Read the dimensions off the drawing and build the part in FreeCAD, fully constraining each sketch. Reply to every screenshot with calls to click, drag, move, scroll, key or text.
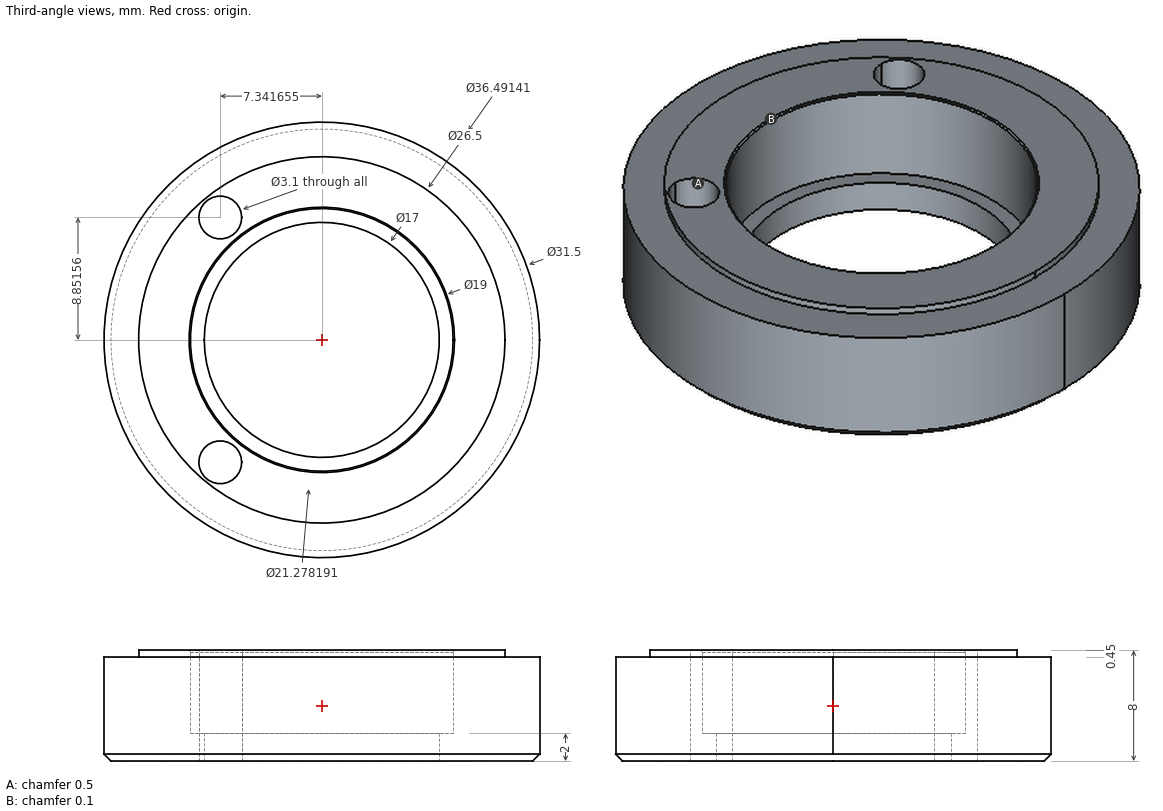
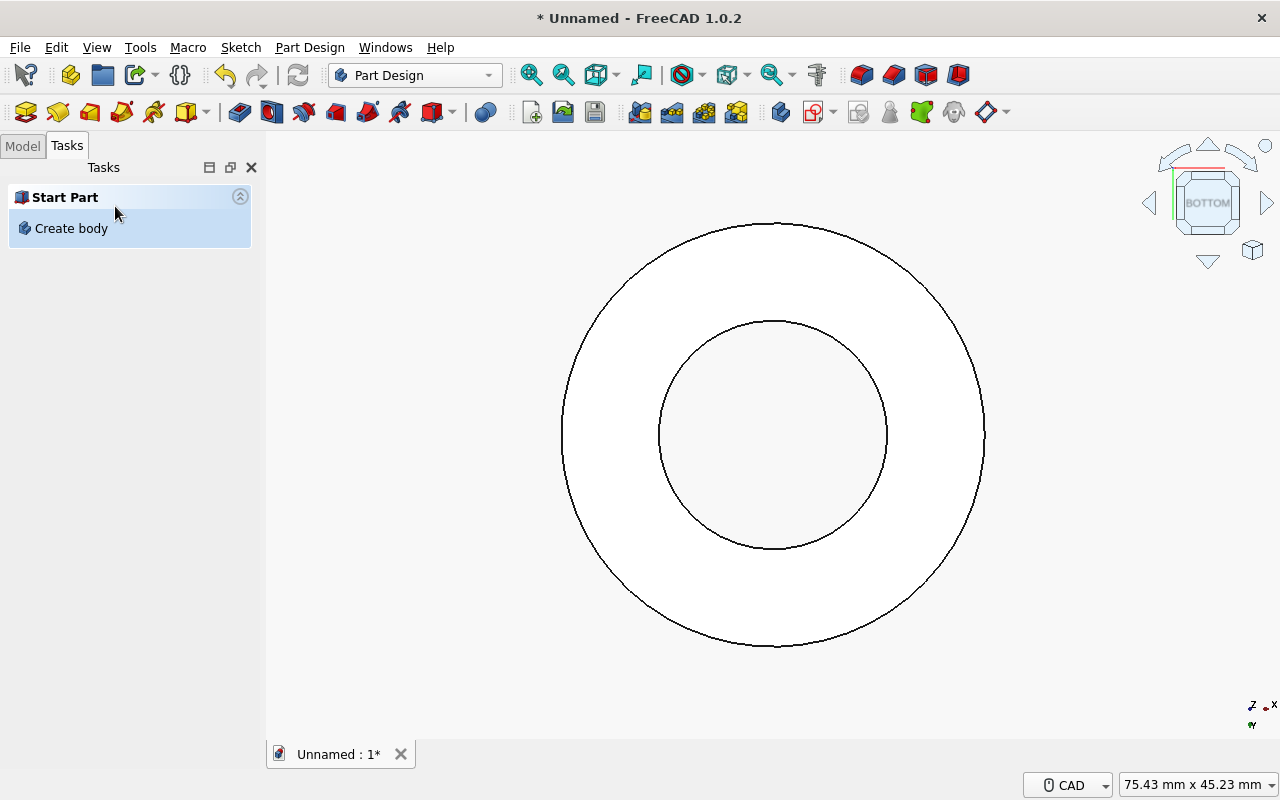
click(652, 313)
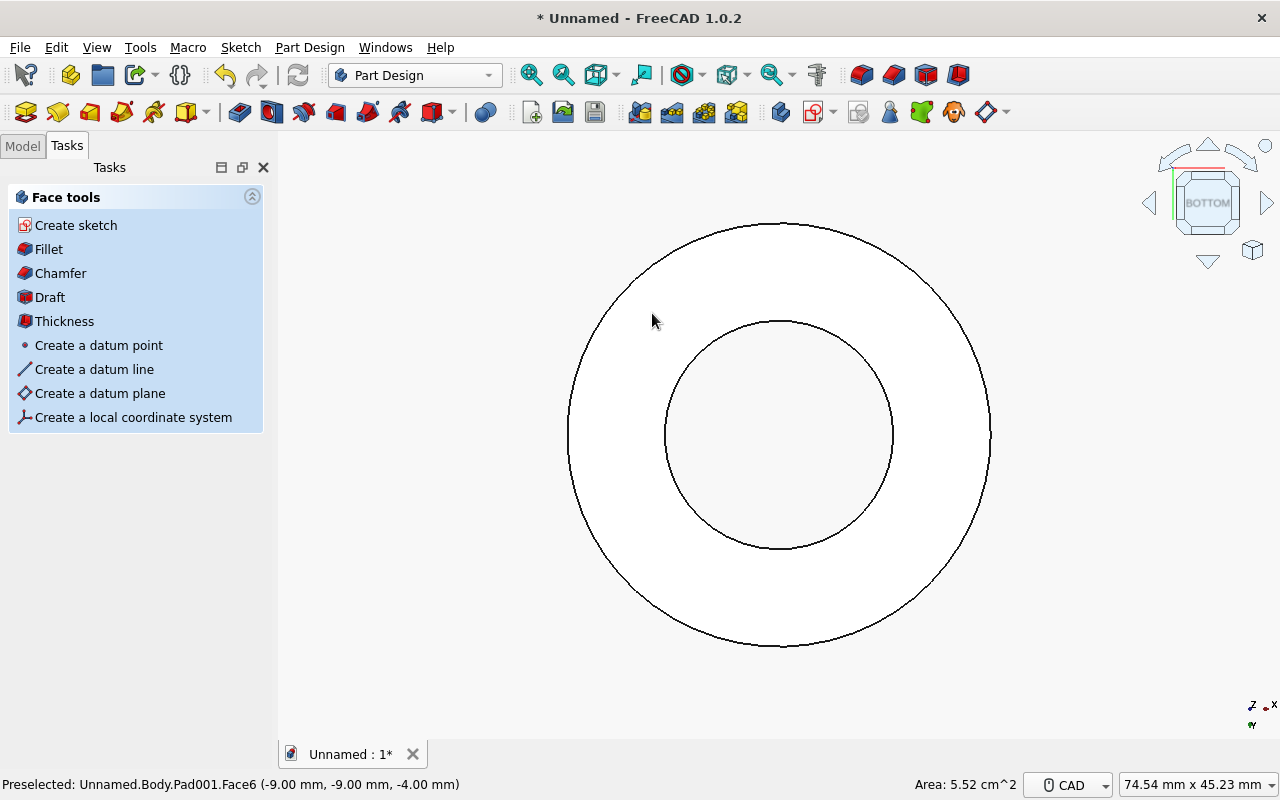
click(814, 112)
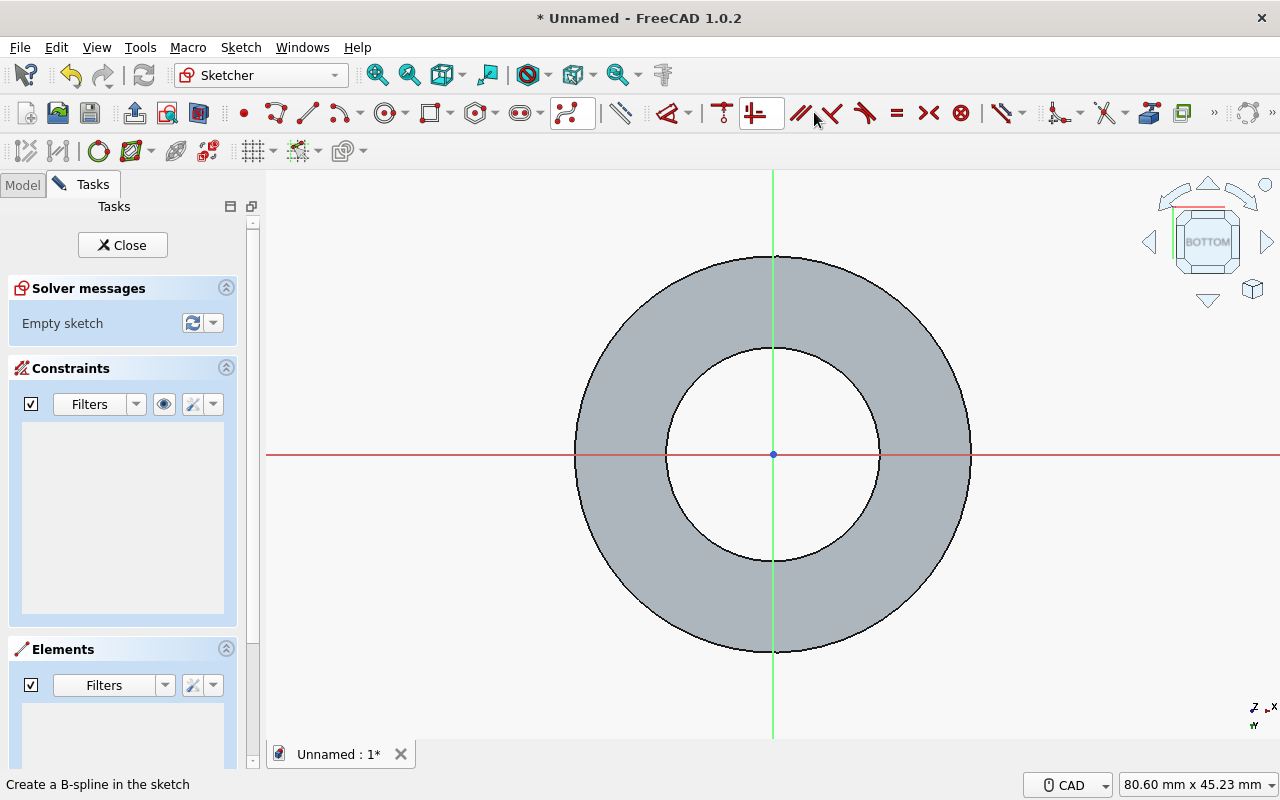
scroll(678, 580, up, 11)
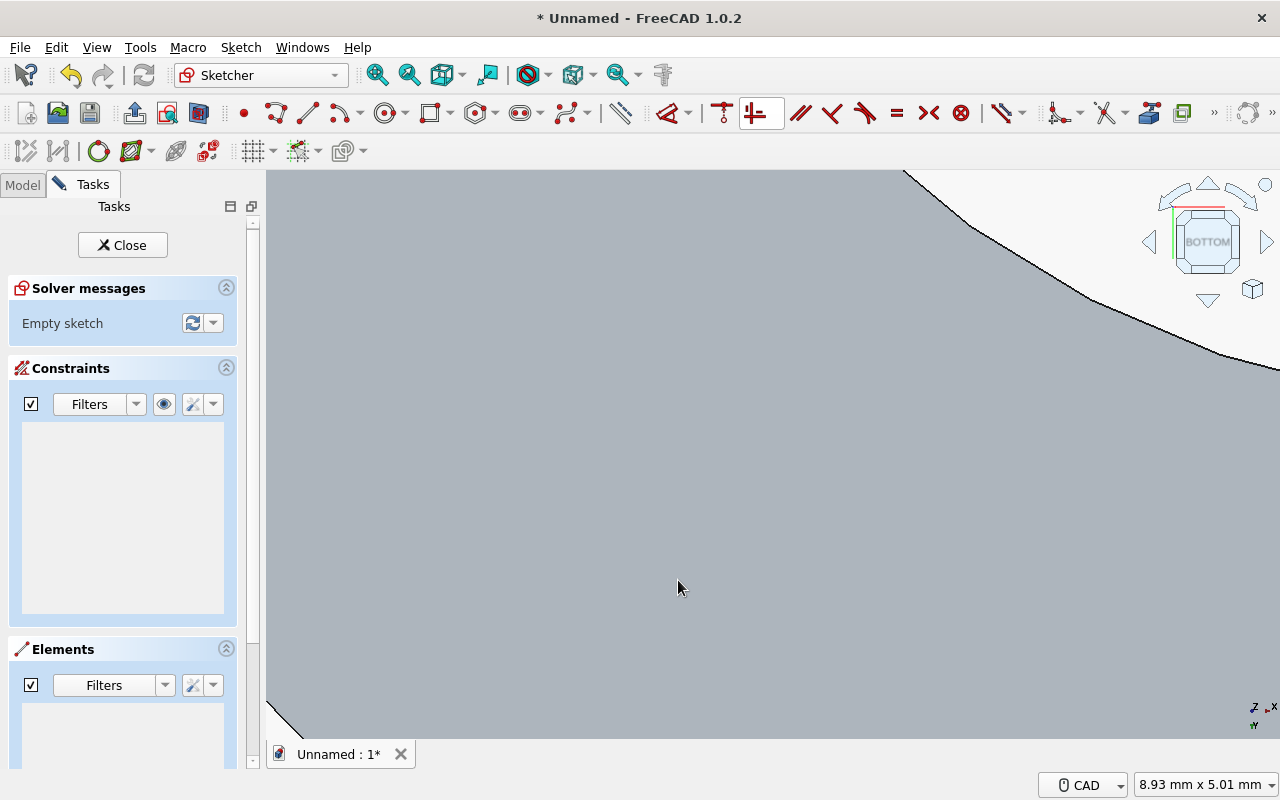
key(g)
key(c)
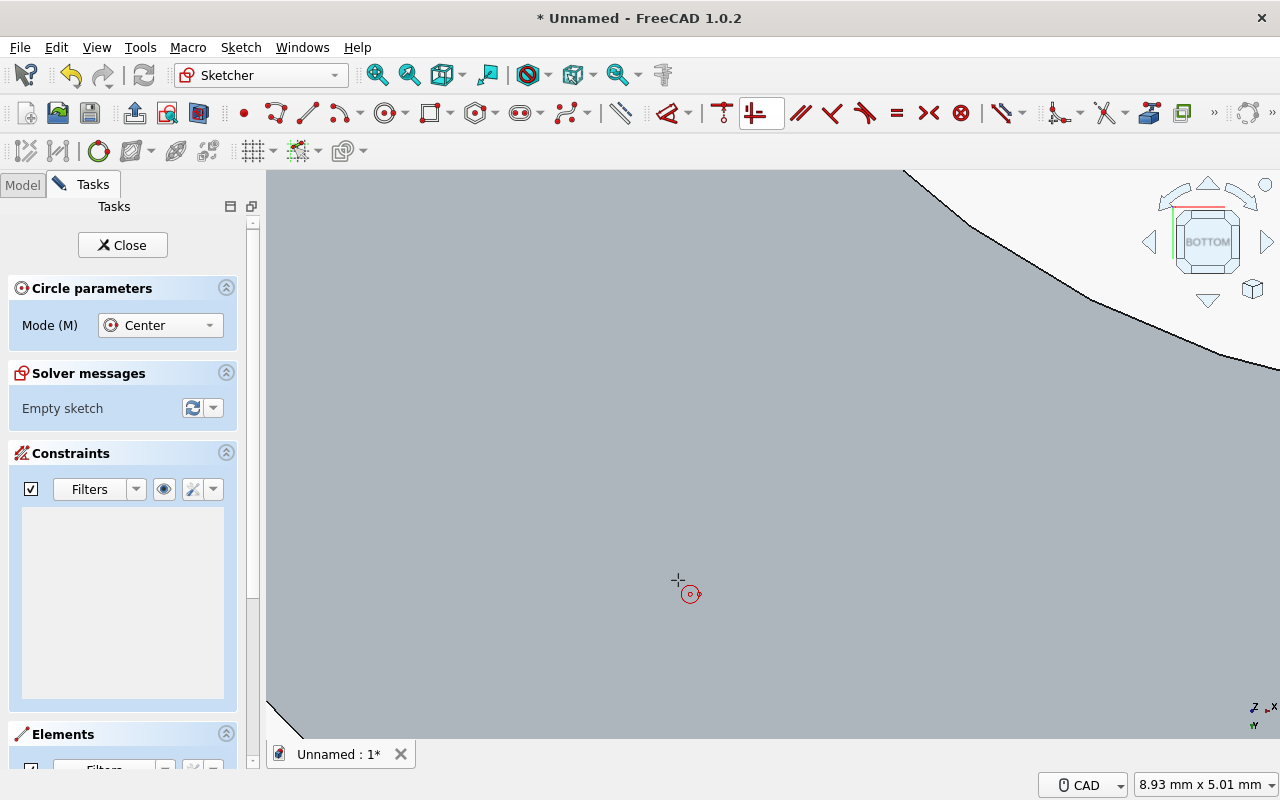
click(699, 447)
move(823, 322)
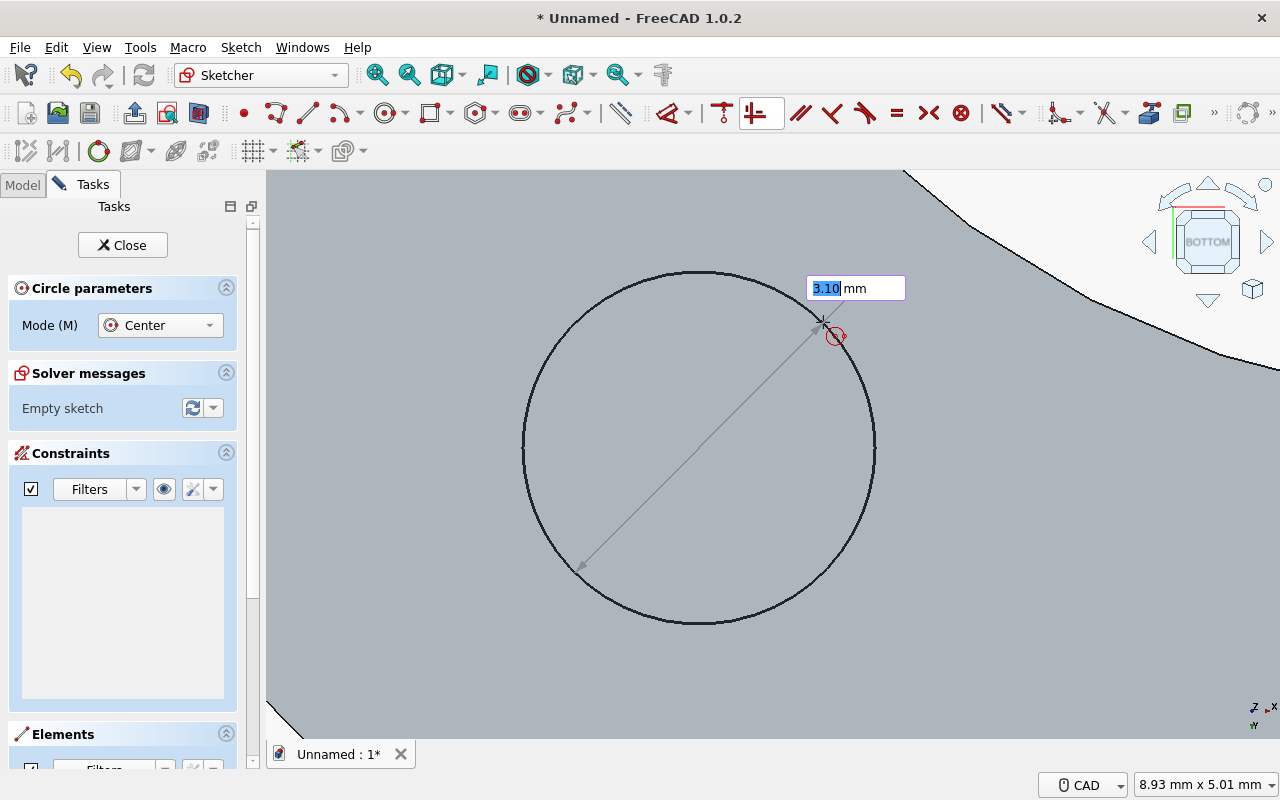
text(3.1)
key(Return)
key(Escape)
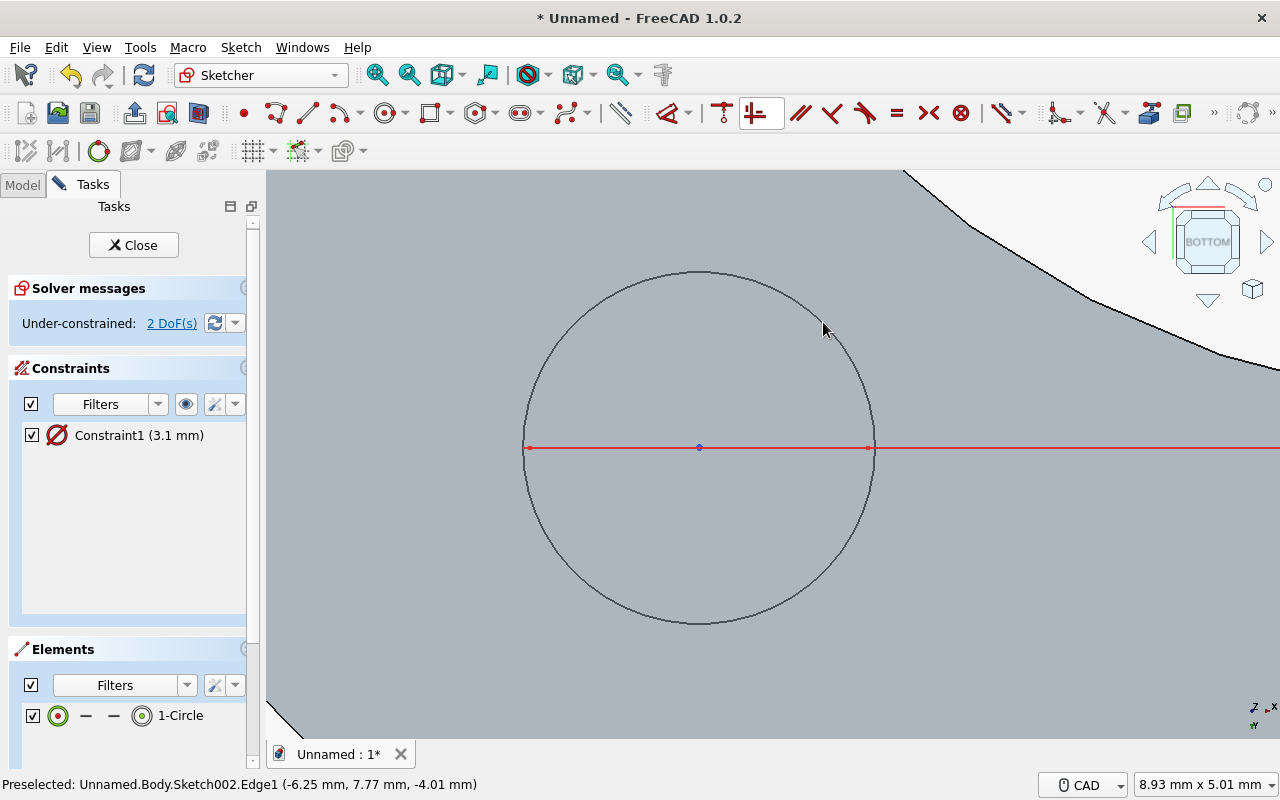
click(668, 114)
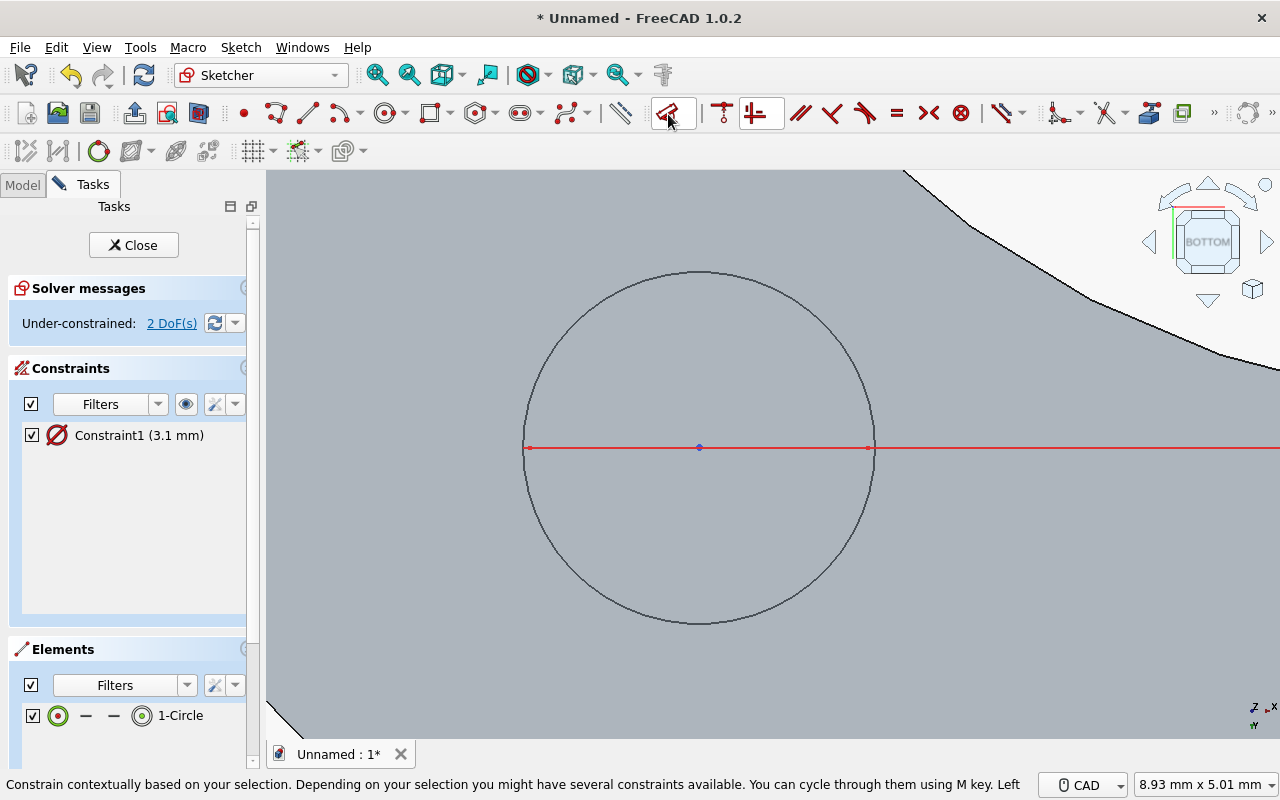
click(699, 448)
click(665, 323)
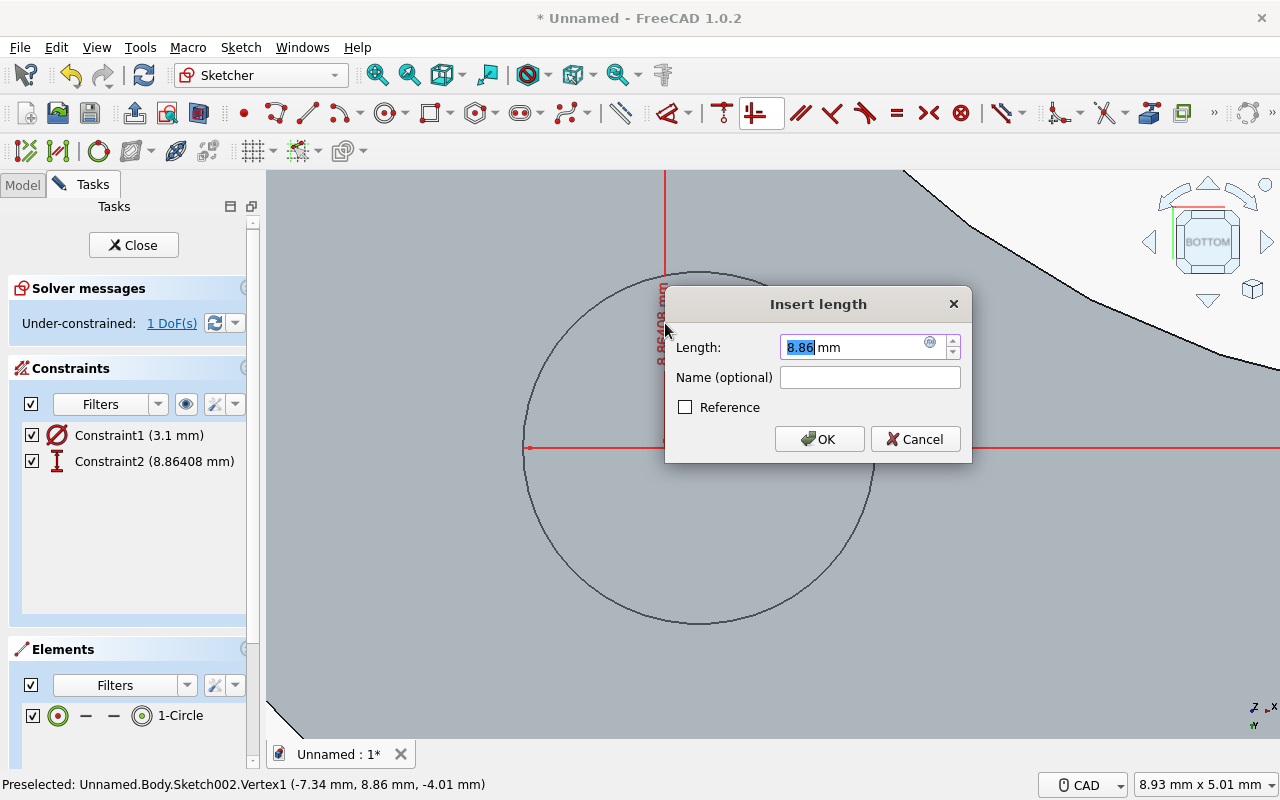
text(8.85156)
key(Return)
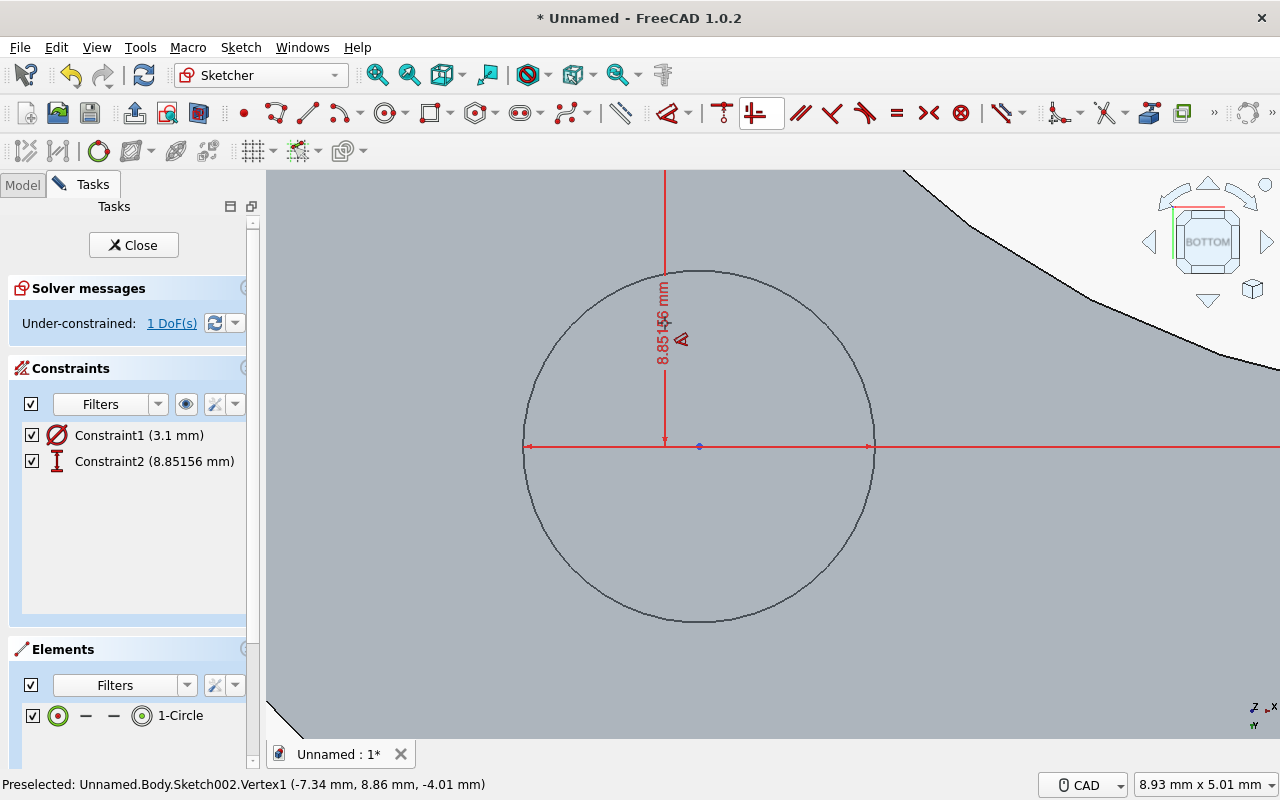
click(699, 447)
click(907, 481)